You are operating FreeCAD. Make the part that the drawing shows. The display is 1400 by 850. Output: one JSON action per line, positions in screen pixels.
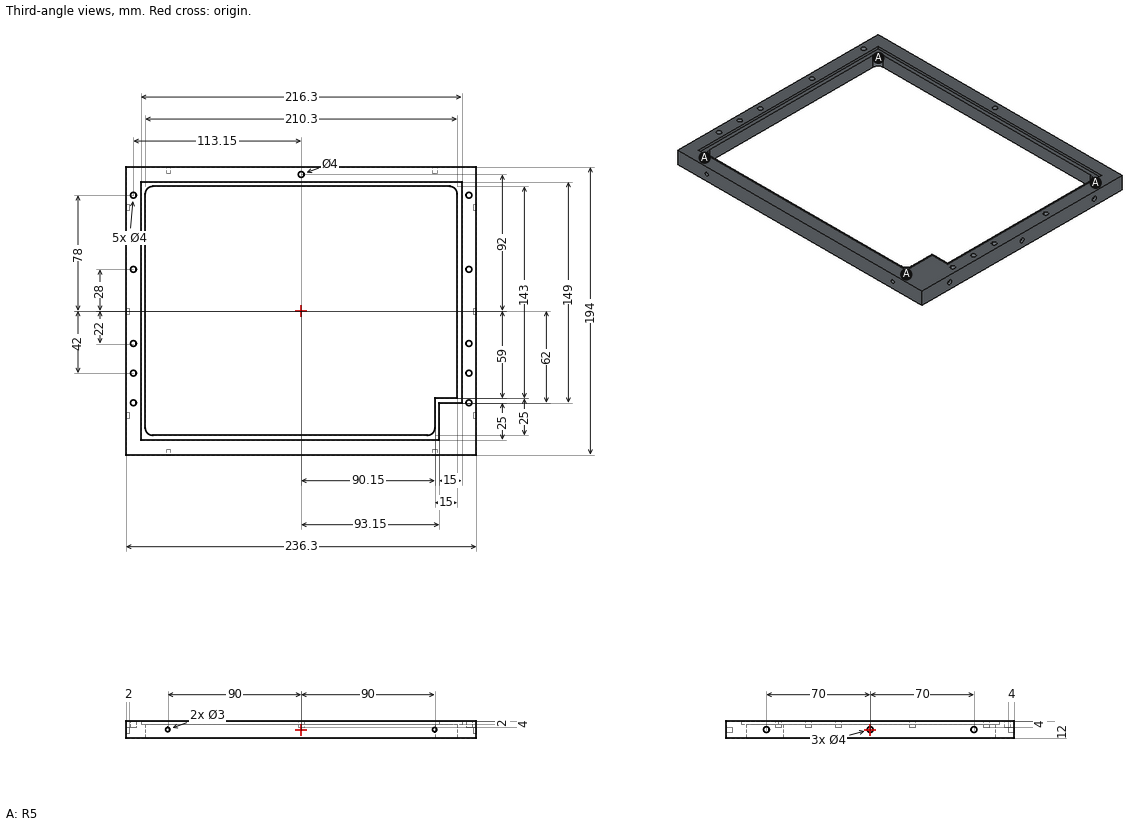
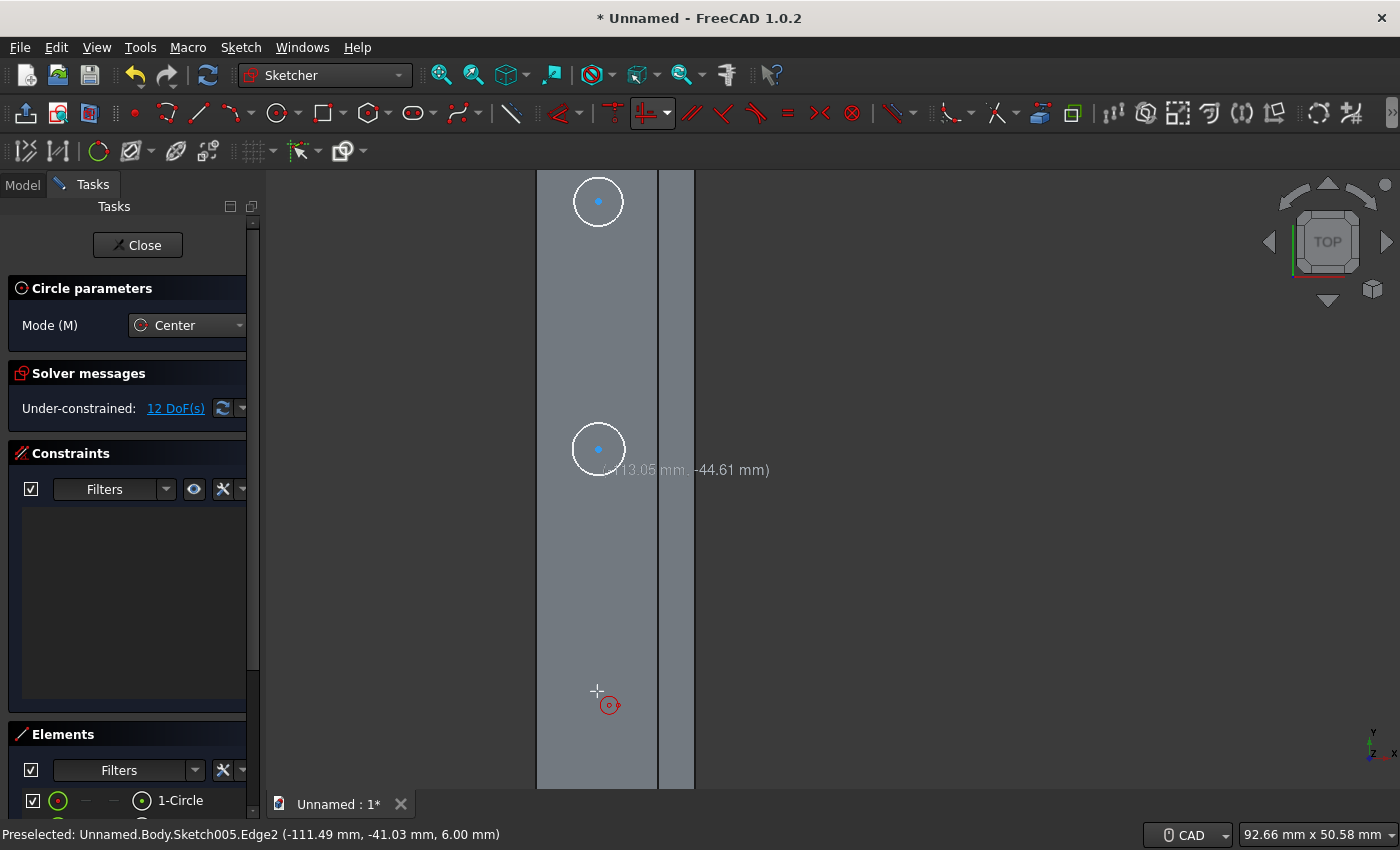
{"action": "scroll", "coordinate": [597, 692], "scroll_direction": "down", "scroll_amount": 7}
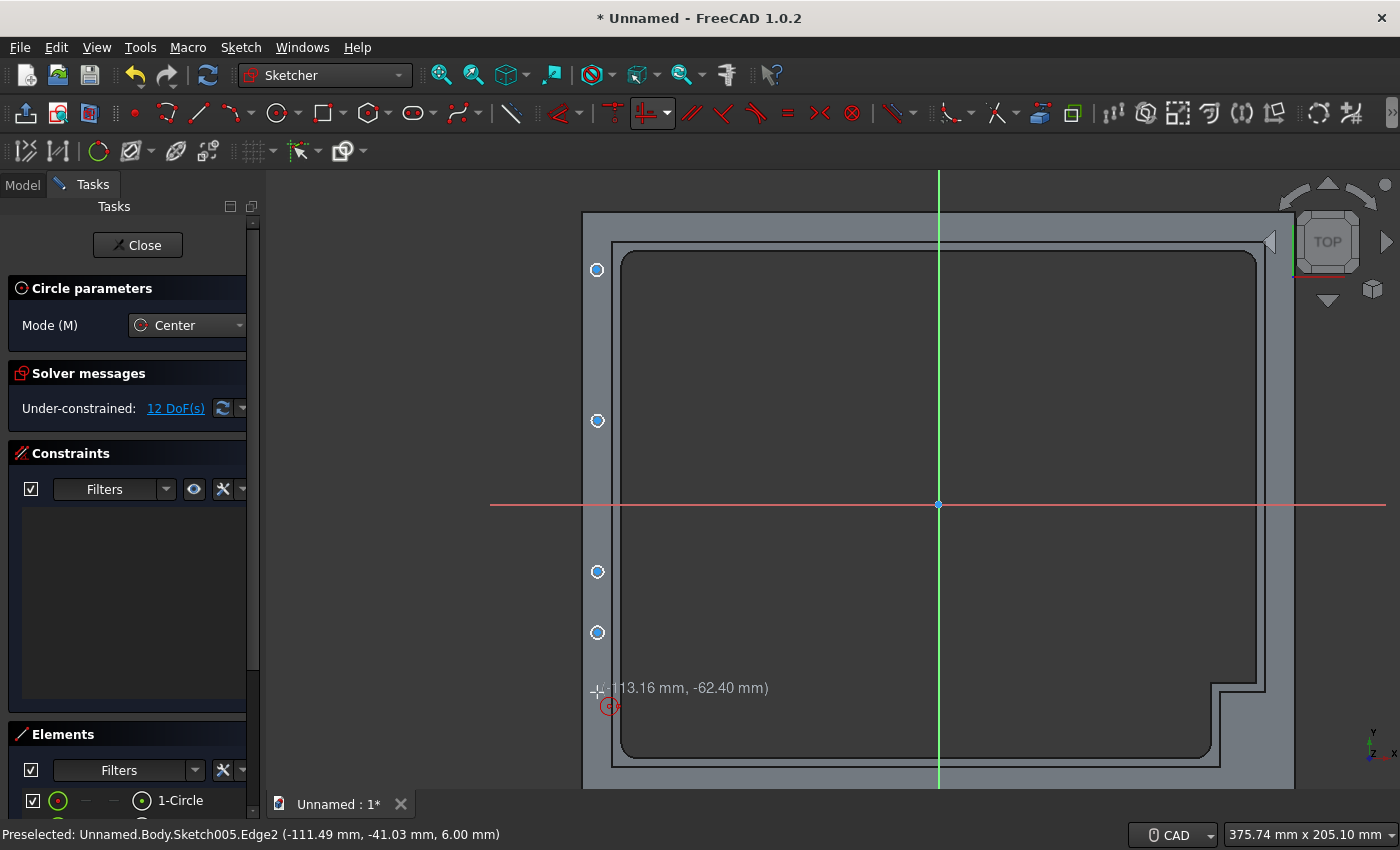
{"action": "left_click", "coordinate": [597, 692]}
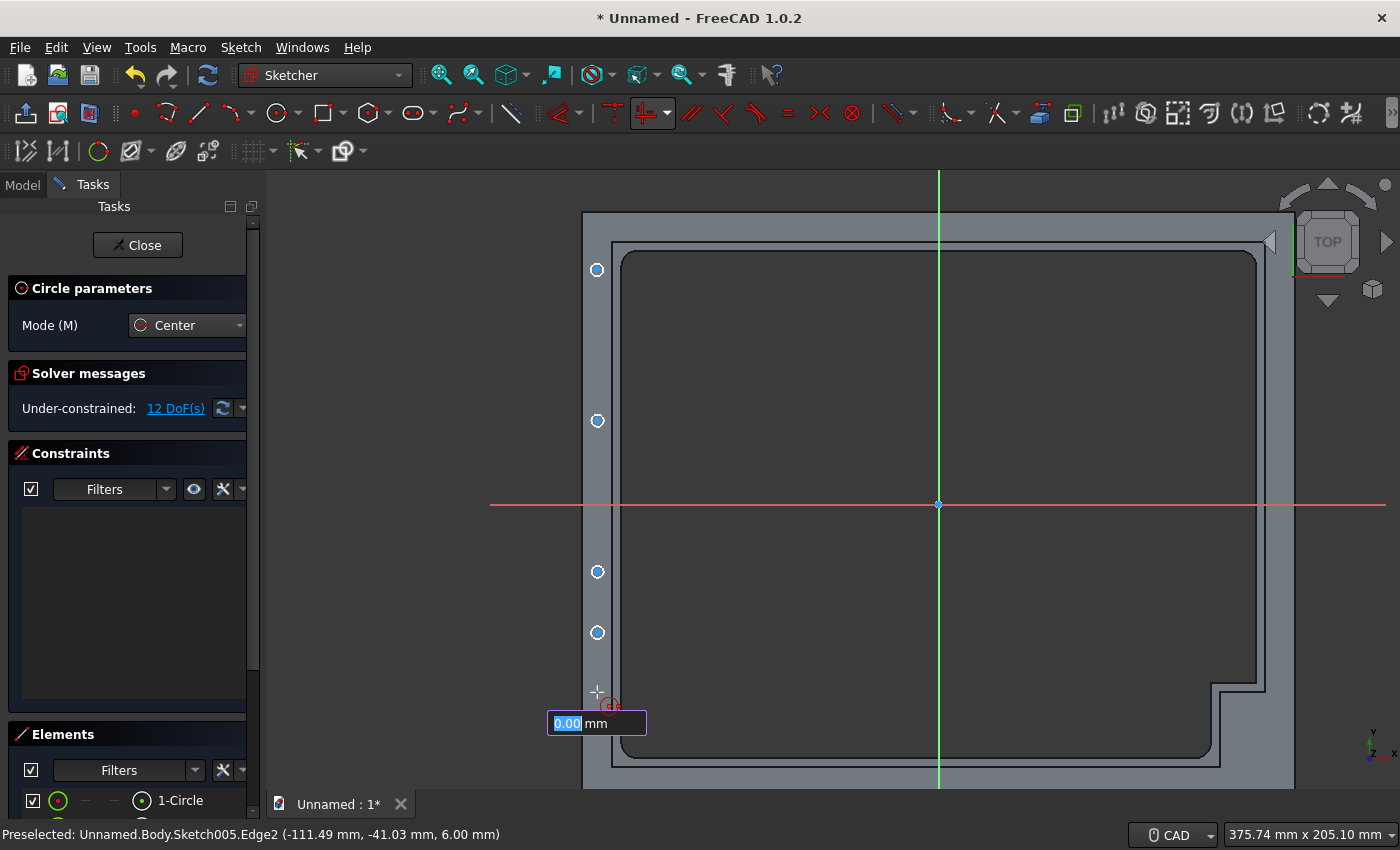
{"action": "scroll", "coordinate": [602, 687], "scroll_direction": "up", "scroll_amount": 5}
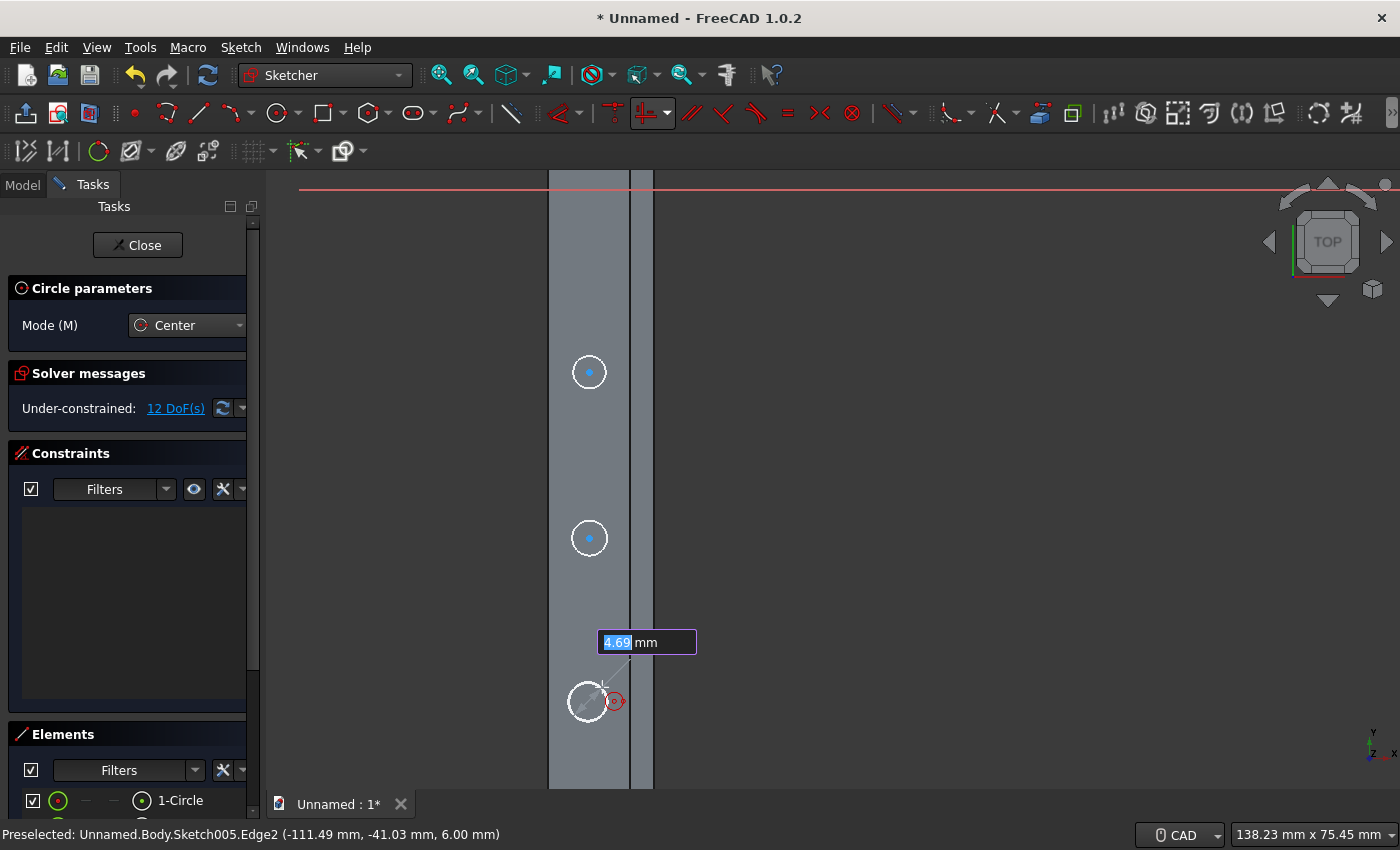
{"action": "left_click", "coordinate": [600, 687]}
{"action": "key", "text": "Escape"}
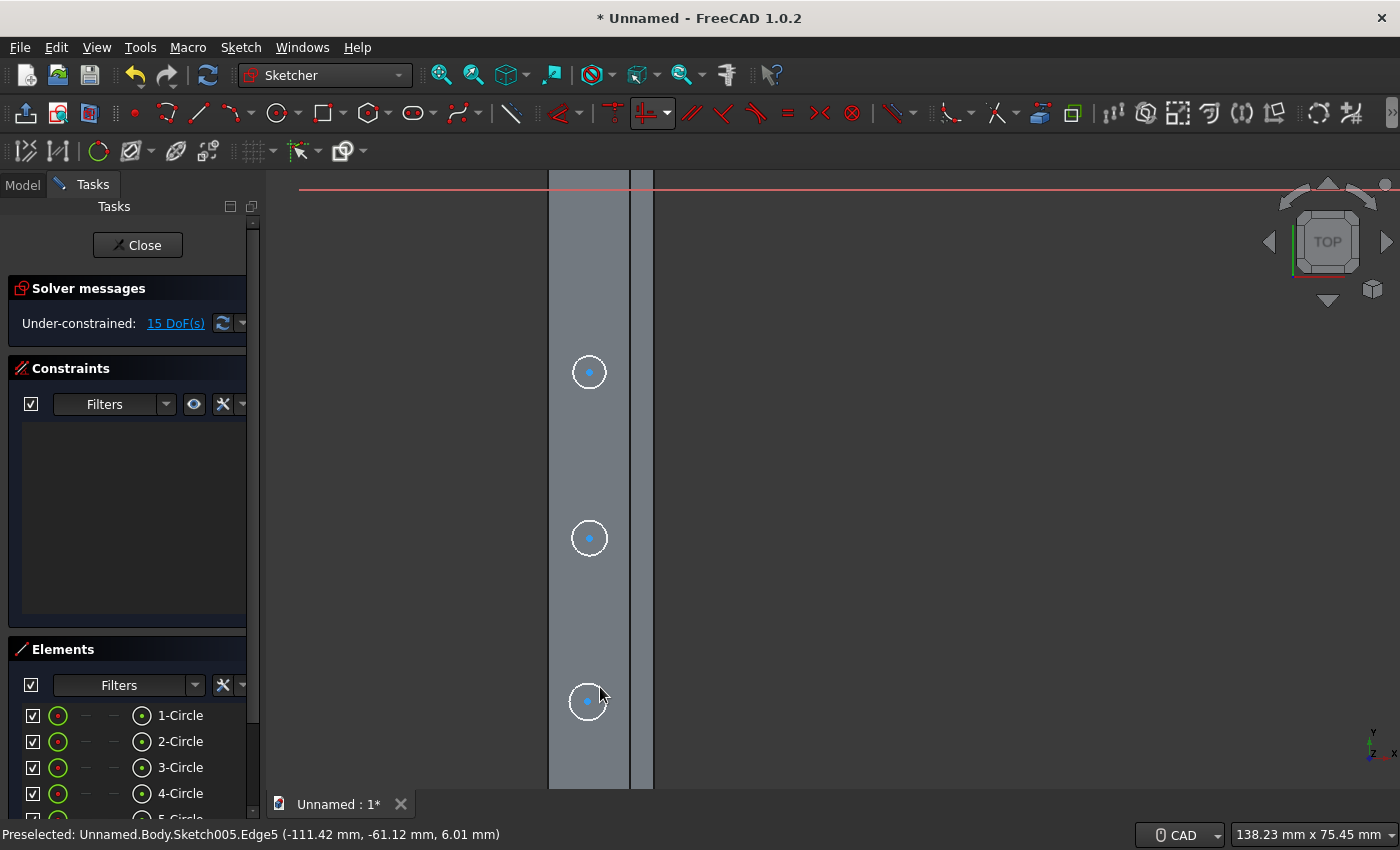
{"action": "scroll", "coordinate": [602, 686], "scroll_direction": "down", "scroll_amount": 5}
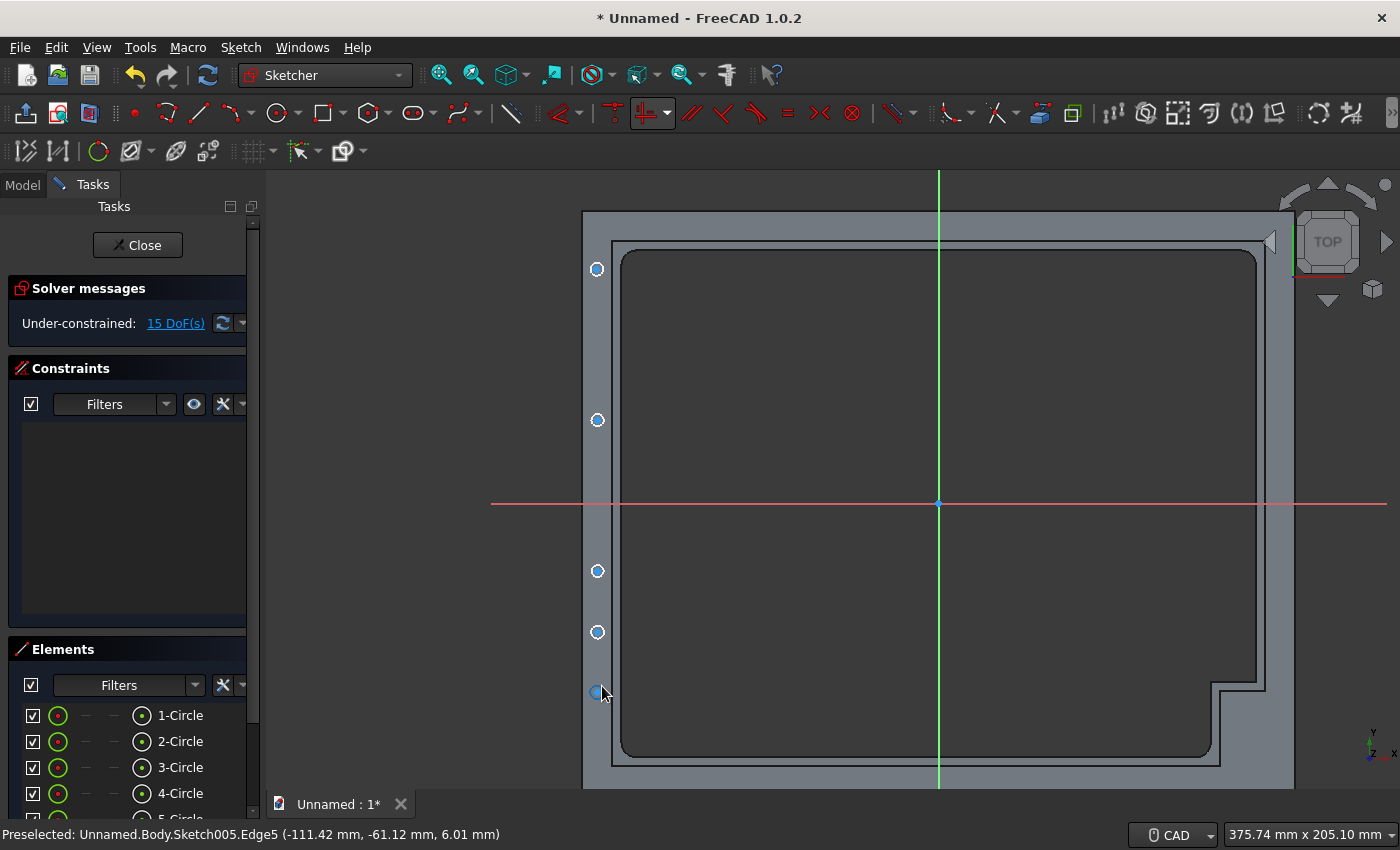
{"action": "scroll", "coordinate": [601, 265], "scroll_direction": "up", "scroll_amount": 4}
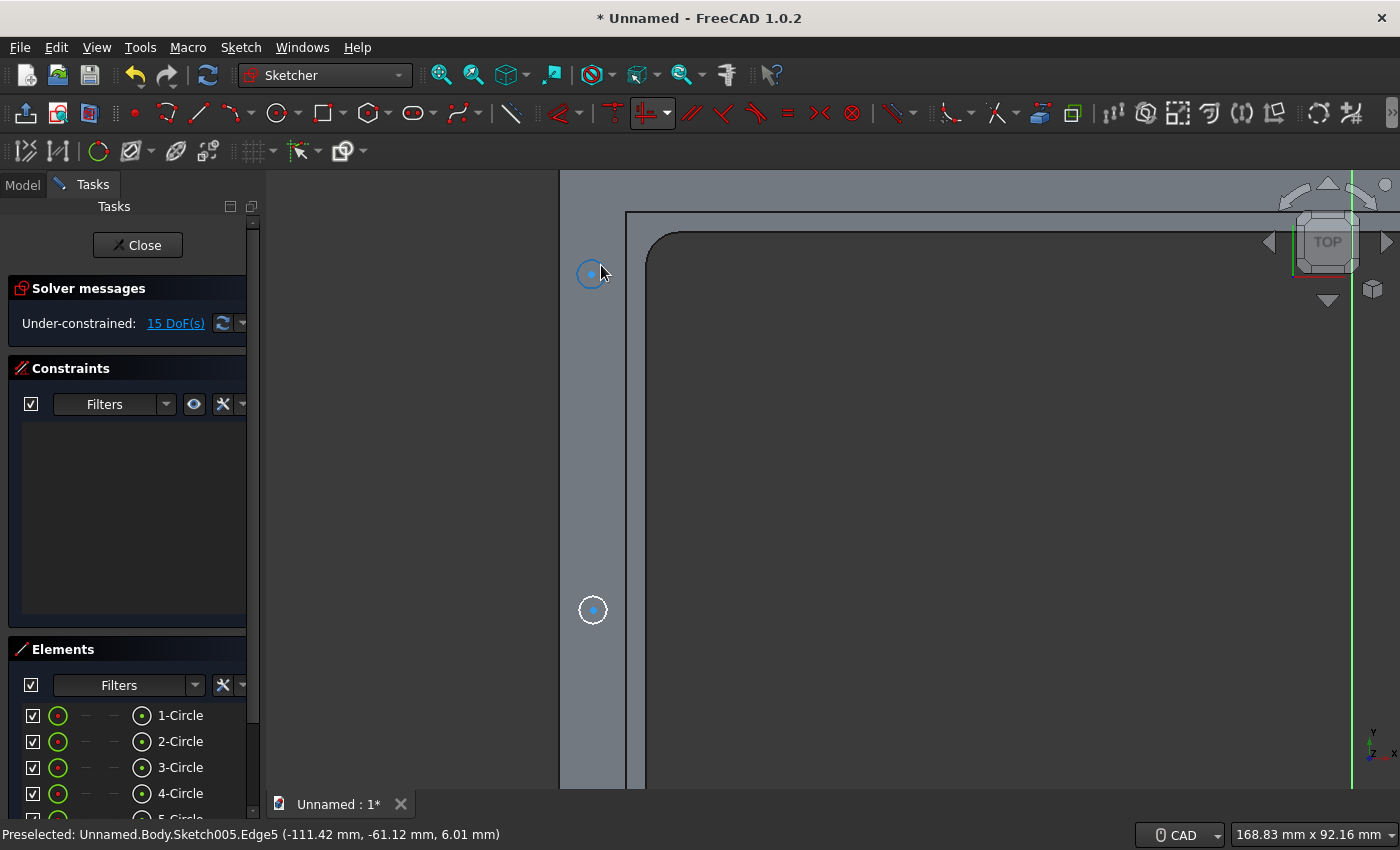
{"action": "left_click", "coordinate": [601, 264]}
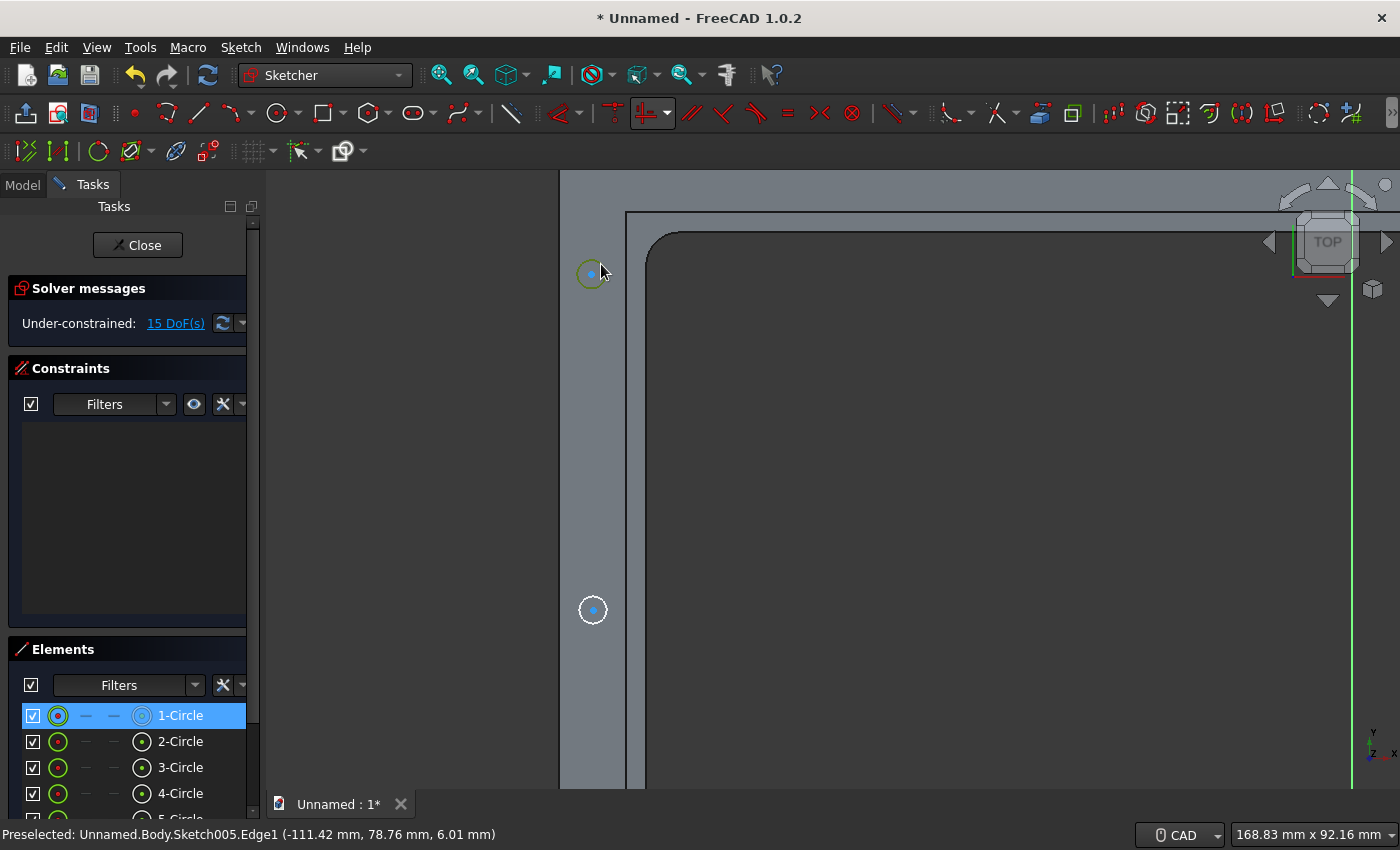
{"action": "left_click", "coordinate": [603, 600]}